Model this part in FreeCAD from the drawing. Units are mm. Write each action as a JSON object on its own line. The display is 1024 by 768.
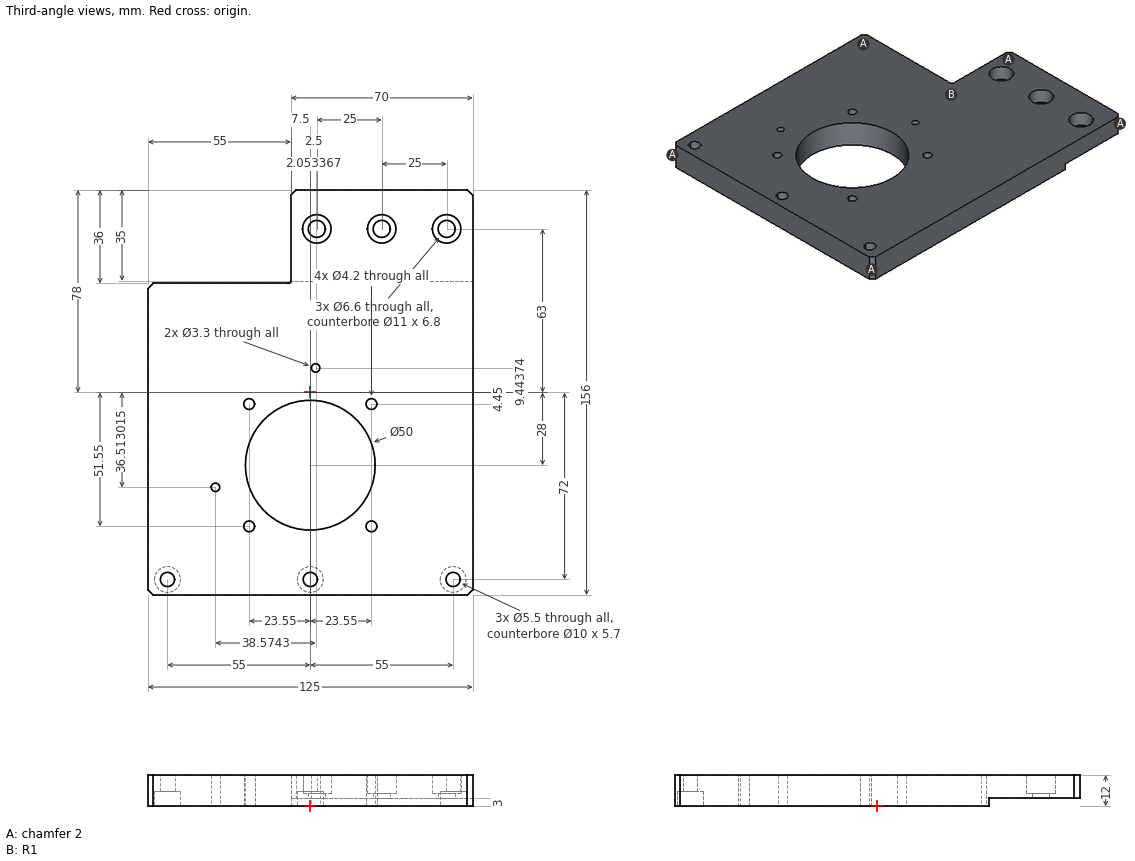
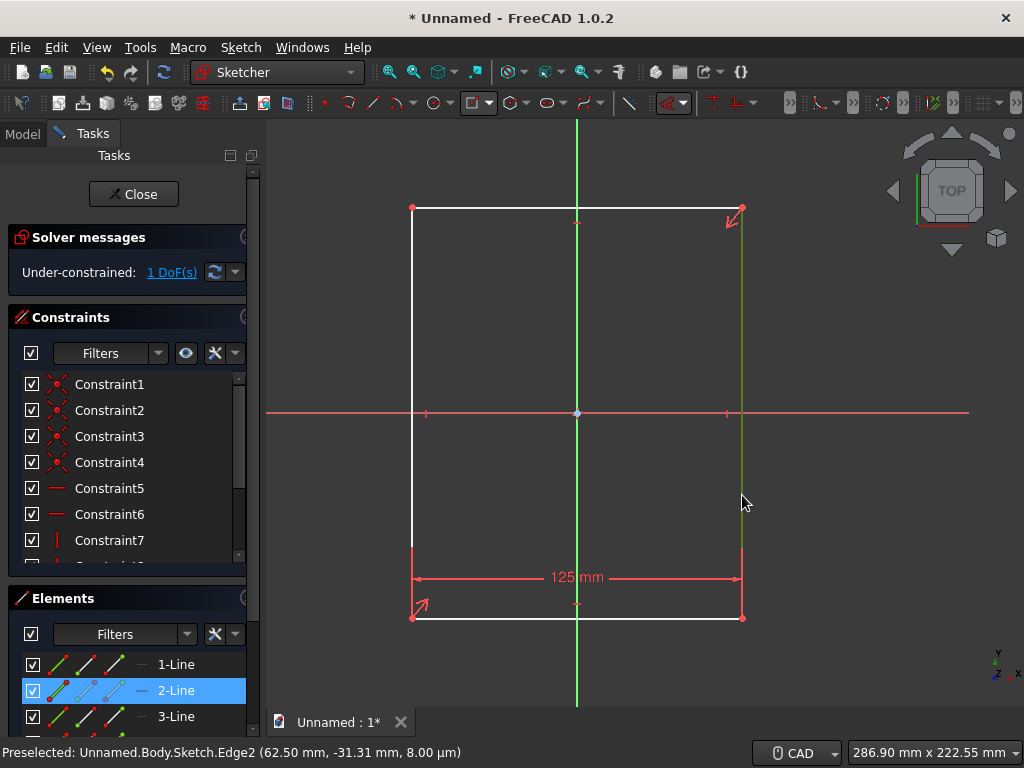
{"action": "key", "text": "i"}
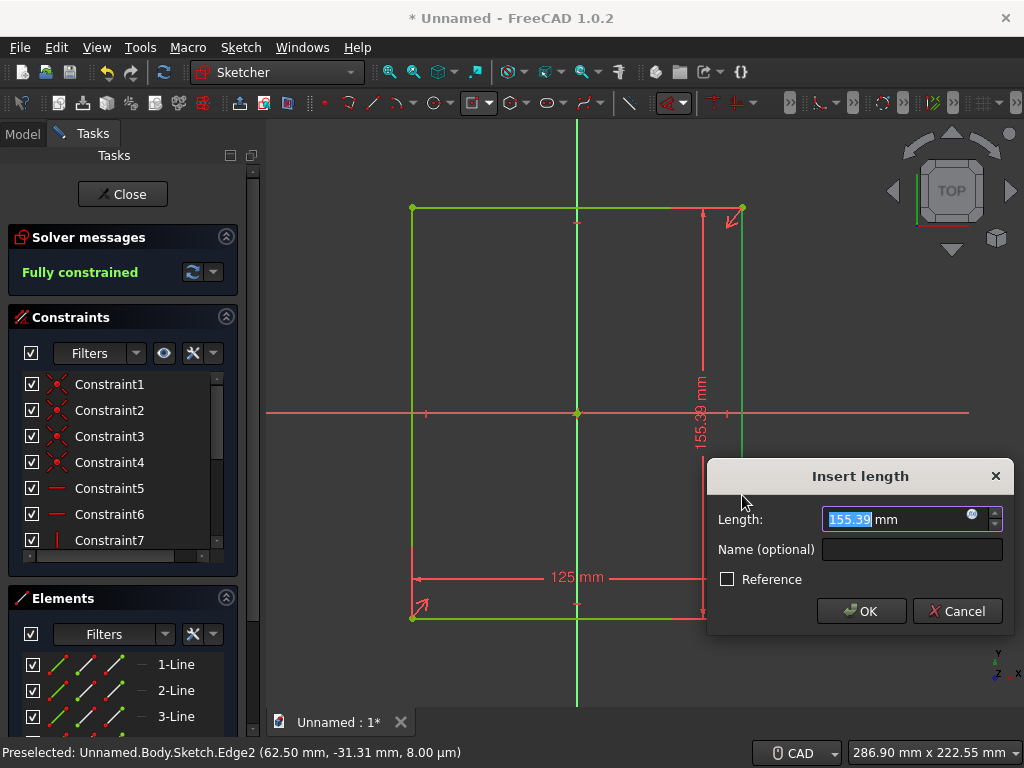
{"action": "type", "text": "156"}
{"action": "key", "text": "Return"}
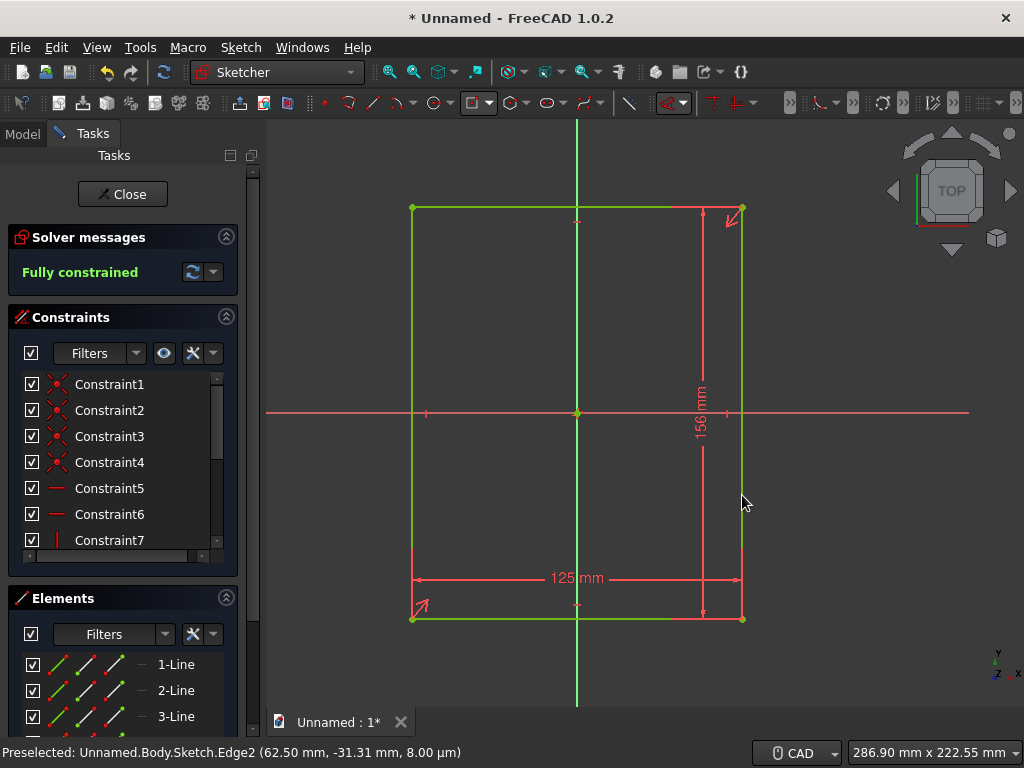
{"action": "left_click", "coordinate": [123, 194]}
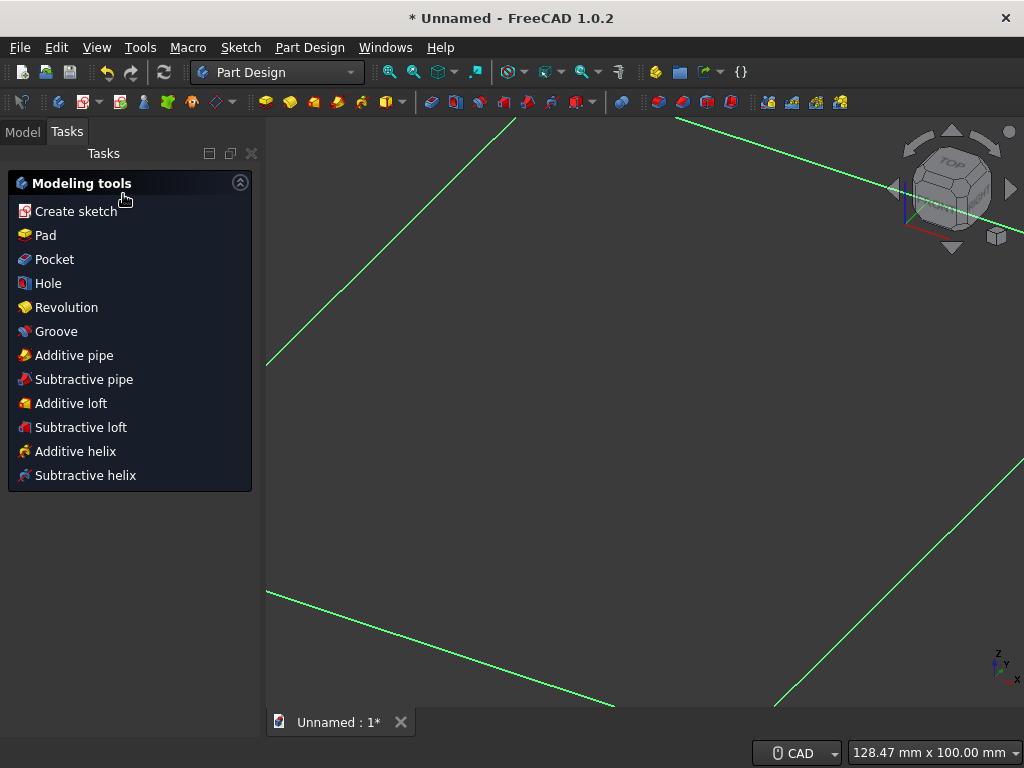
{"action": "left_click", "coordinate": [266, 102]}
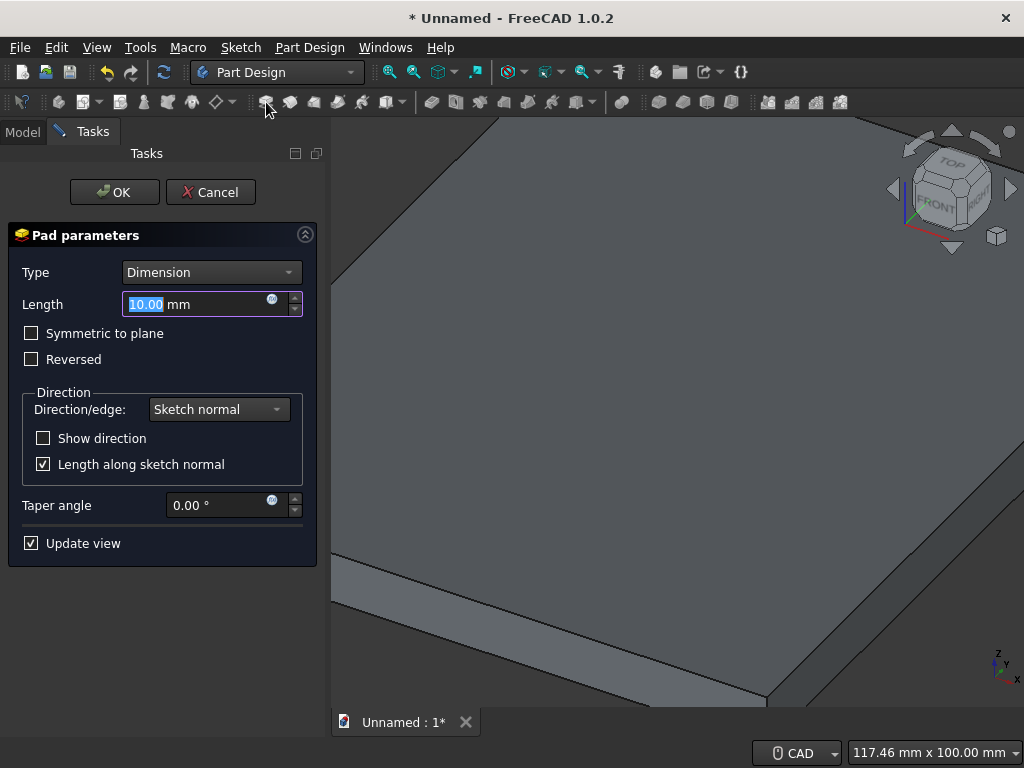
{"action": "type", "text": "12"}
{"action": "key", "text": "Tab"}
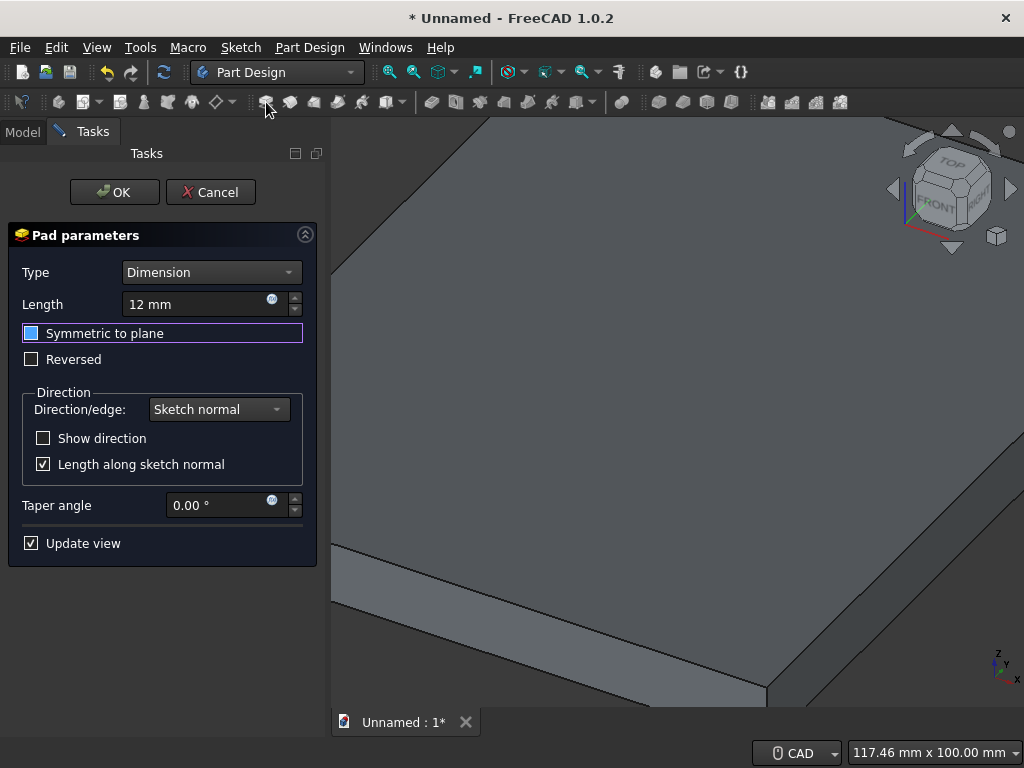
{"action": "left_click", "coordinate": [115, 192]}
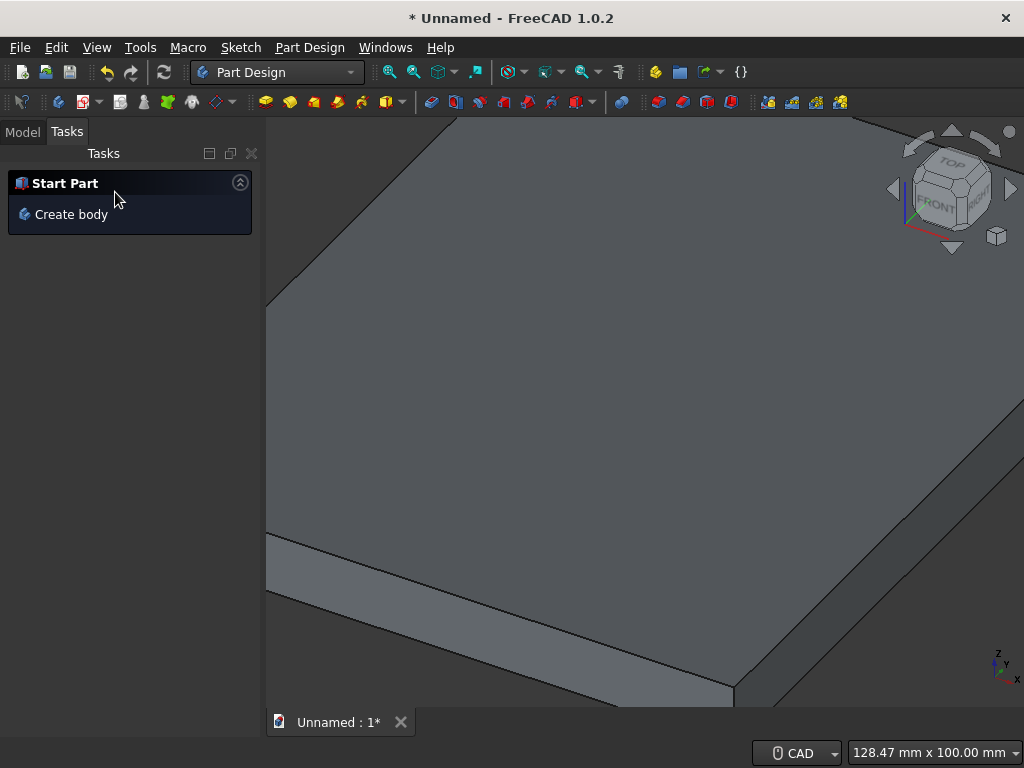
{"action": "left_click", "coordinate": [390, 72]}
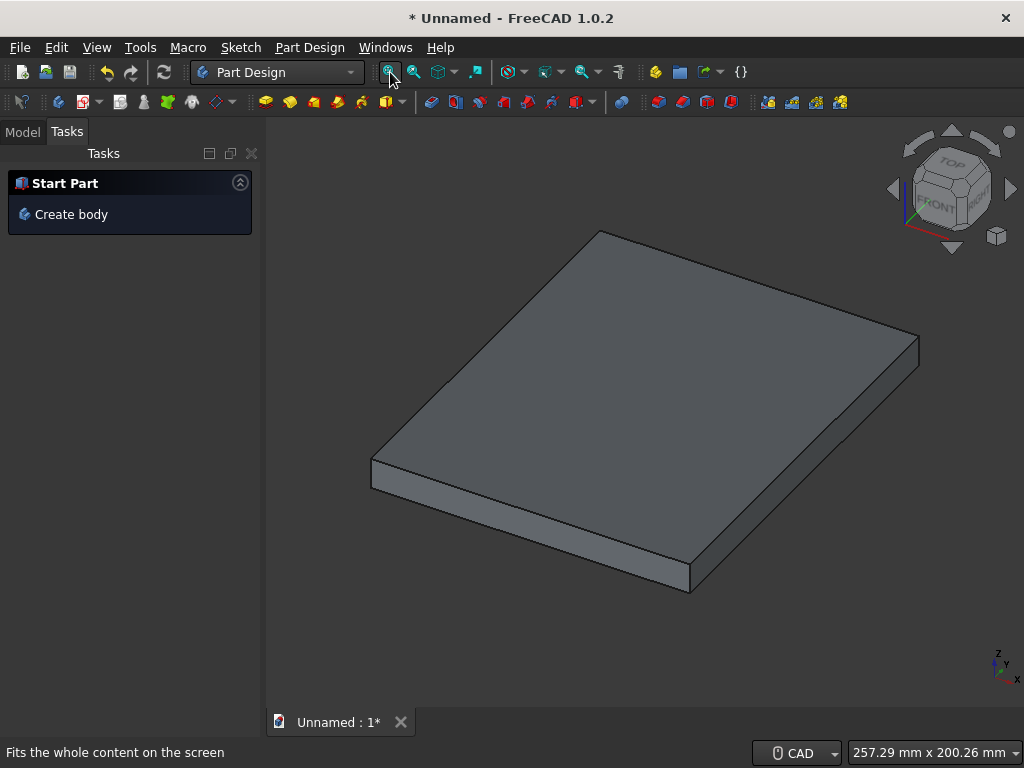
{"action": "left_click", "coordinate": [645, 397]}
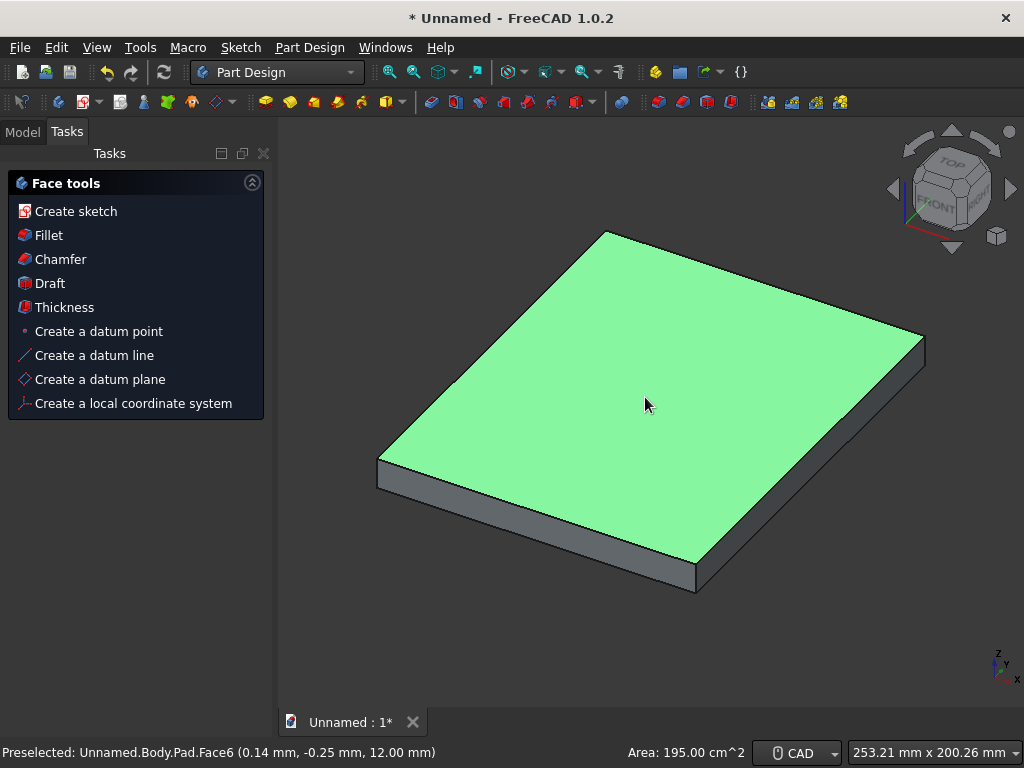
{"action": "left_click", "coordinate": [84, 102]}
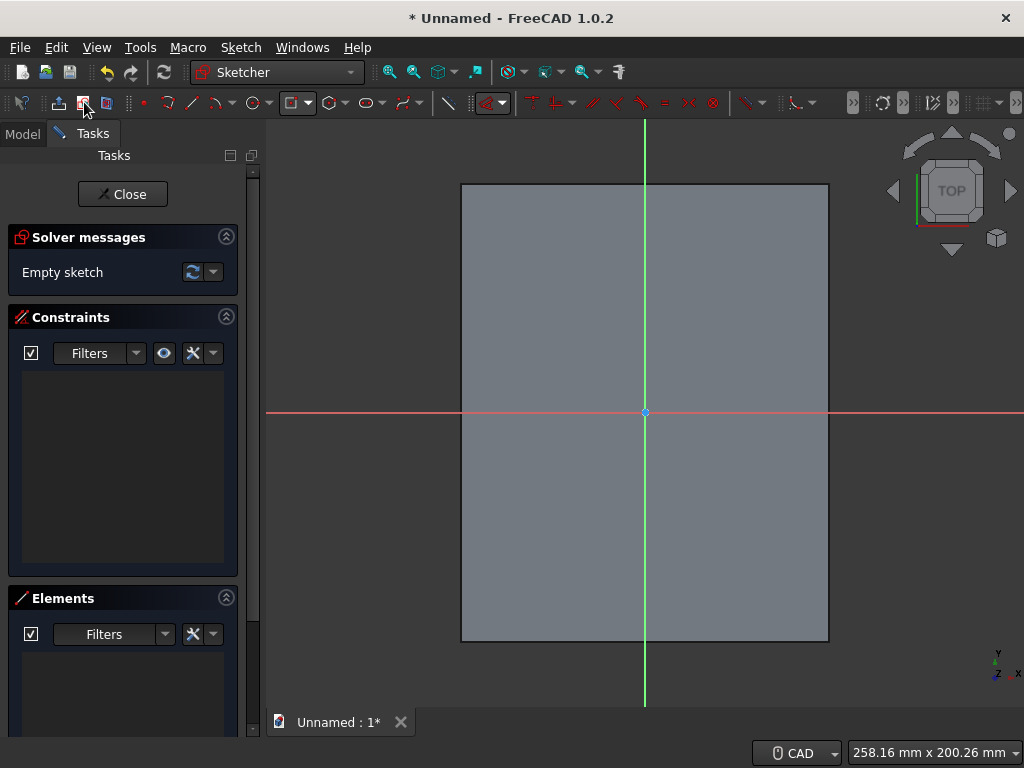
{"action": "scroll", "coordinate": [506, 147], "scroll_direction": "up", "scroll_amount": 2}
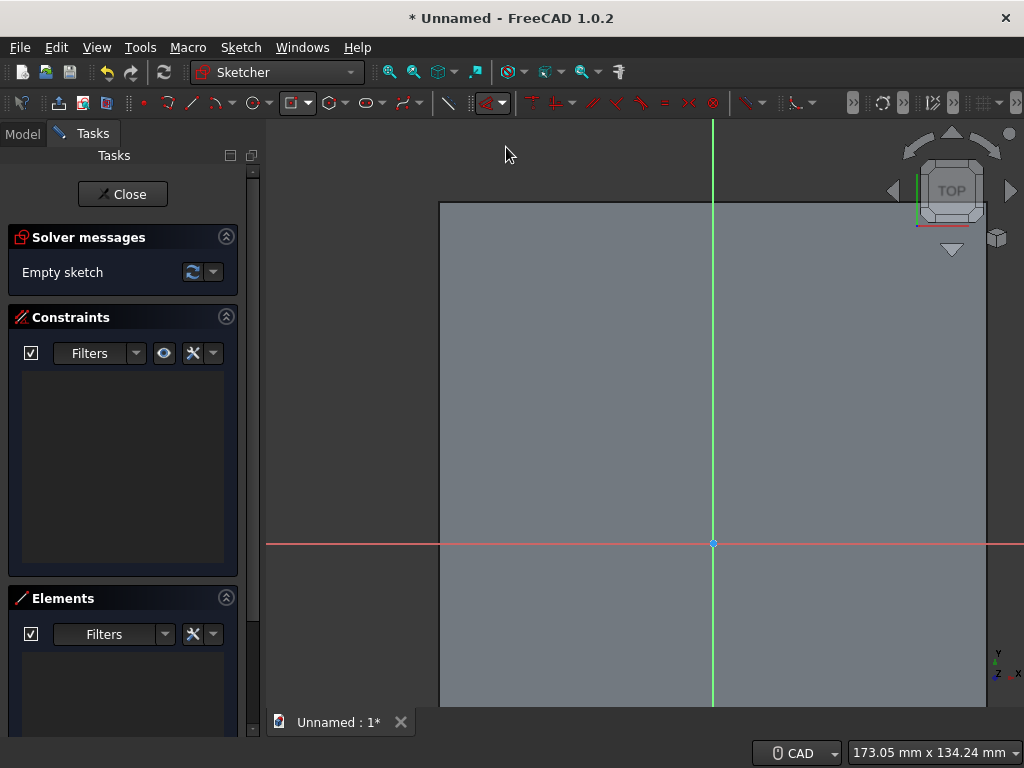
{"action": "left_click", "coordinate": [310, 104]}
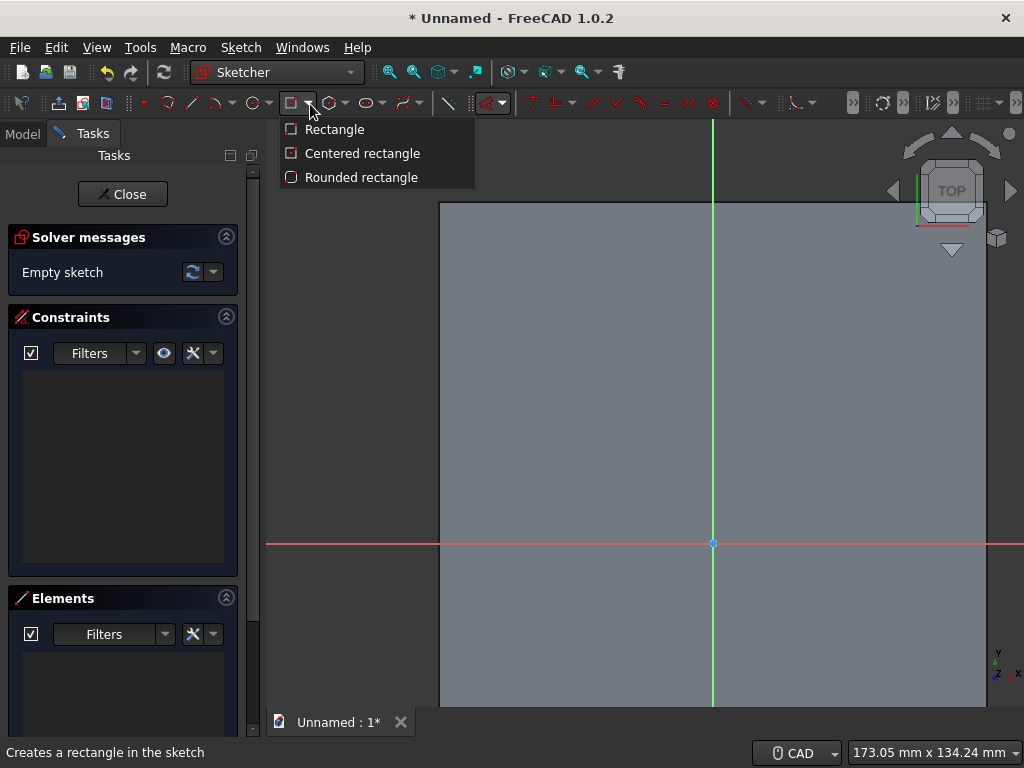
{"action": "left_click", "coordinate": [378, 129]}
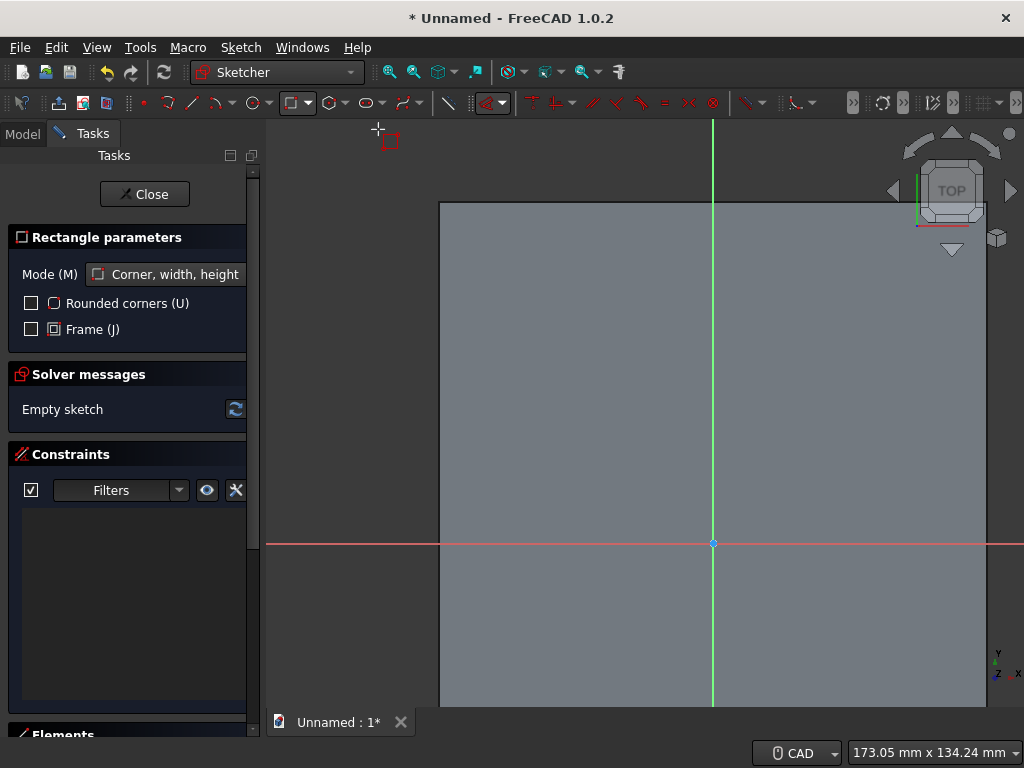
{"action": "left_click", "coordinate": [439, 202]}
{"action": "left_click", "coordinate": [680, 360]}
{"action": "key", "text": "Escape"}